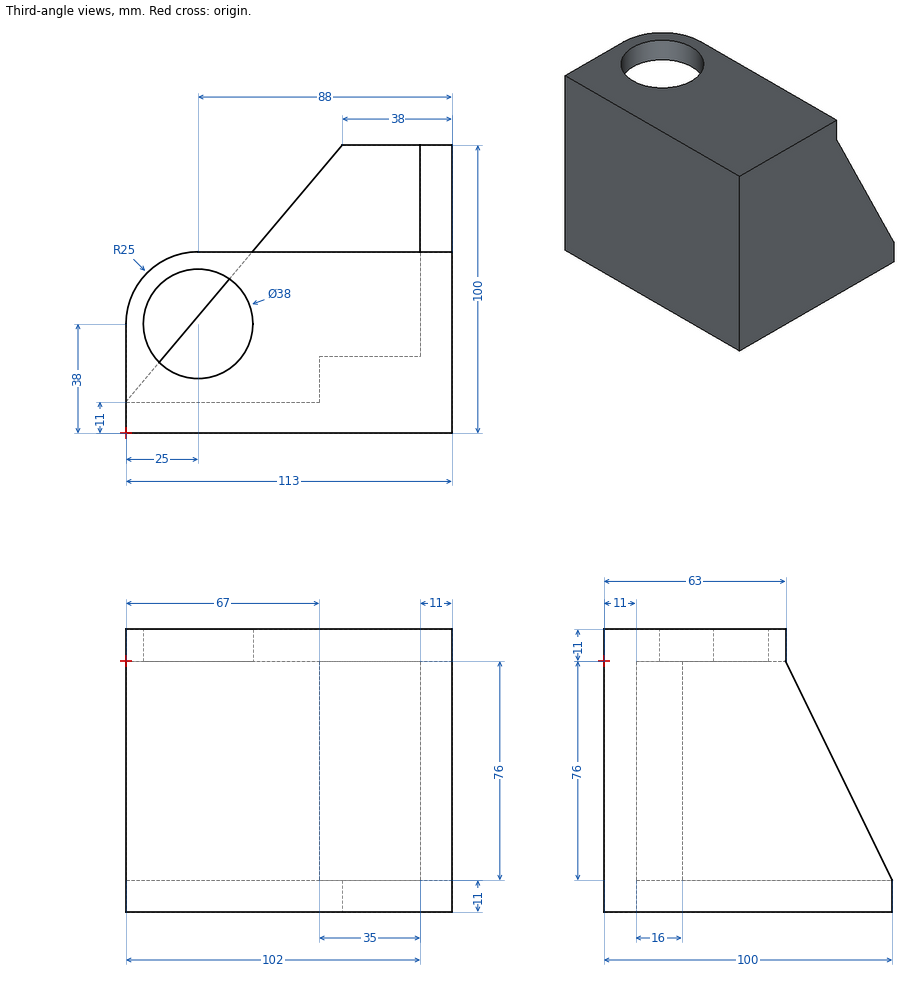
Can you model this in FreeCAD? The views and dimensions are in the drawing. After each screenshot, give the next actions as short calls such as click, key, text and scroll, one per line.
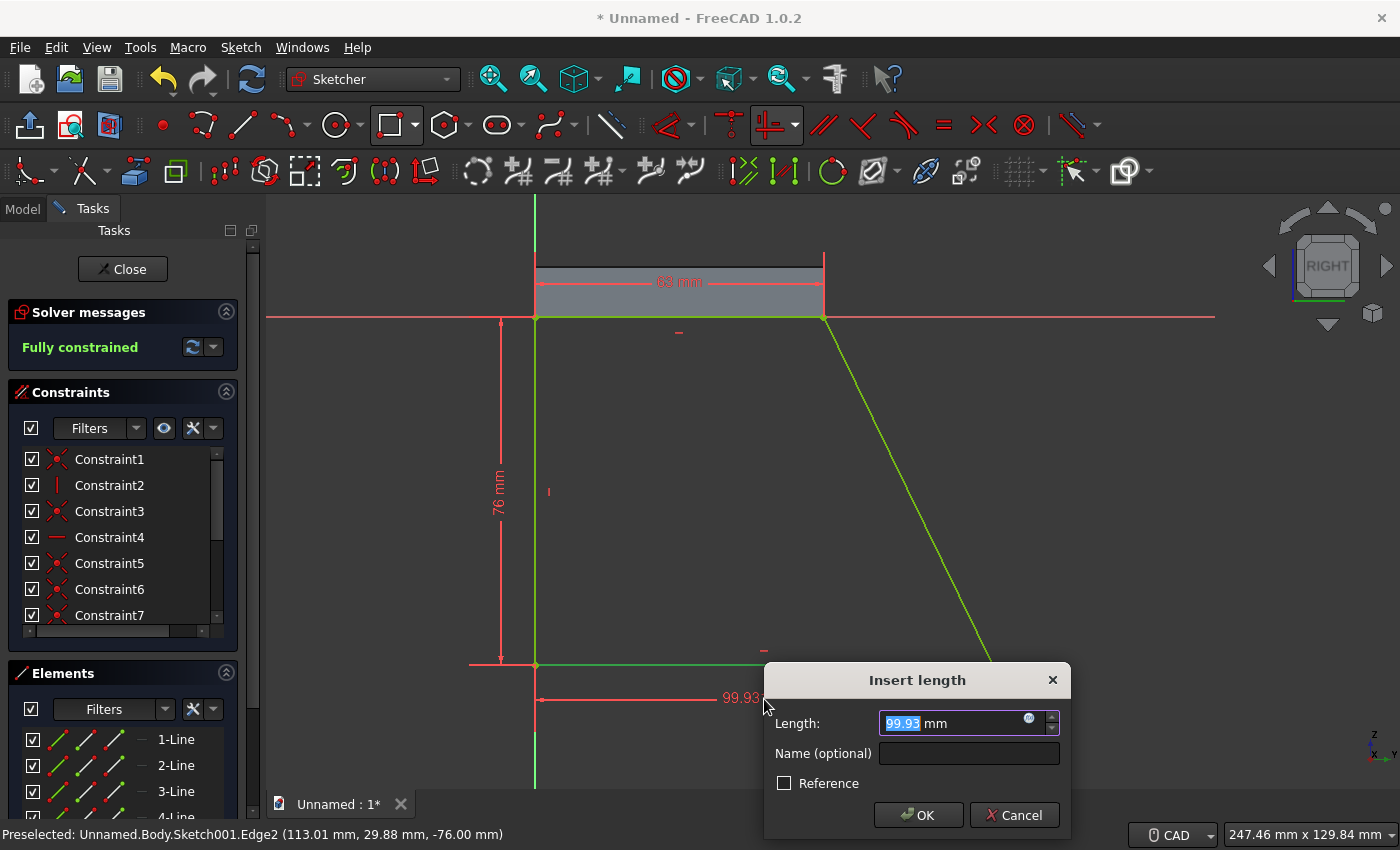
text(100)
key(Return)
key(Escape)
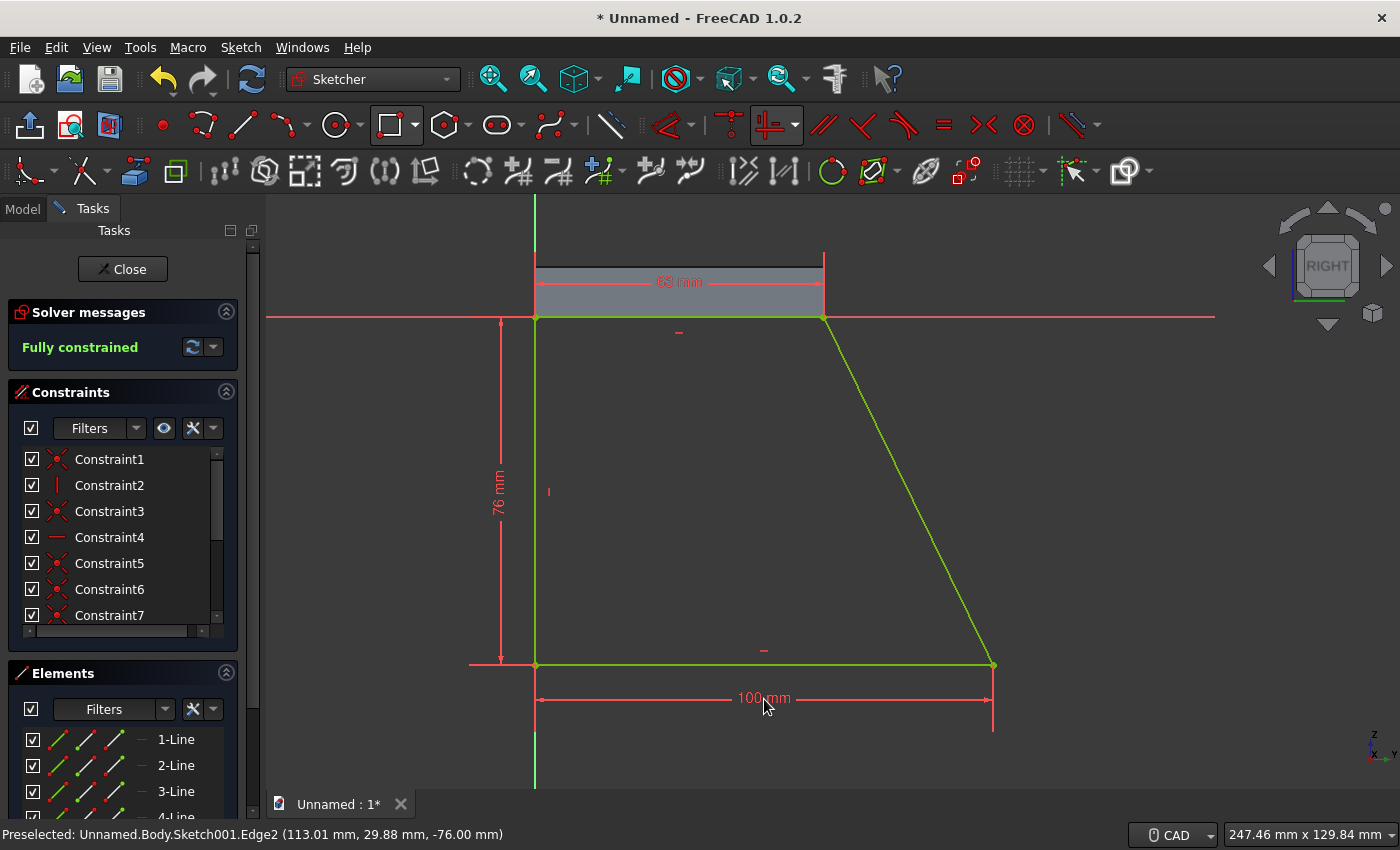
click(123, 269)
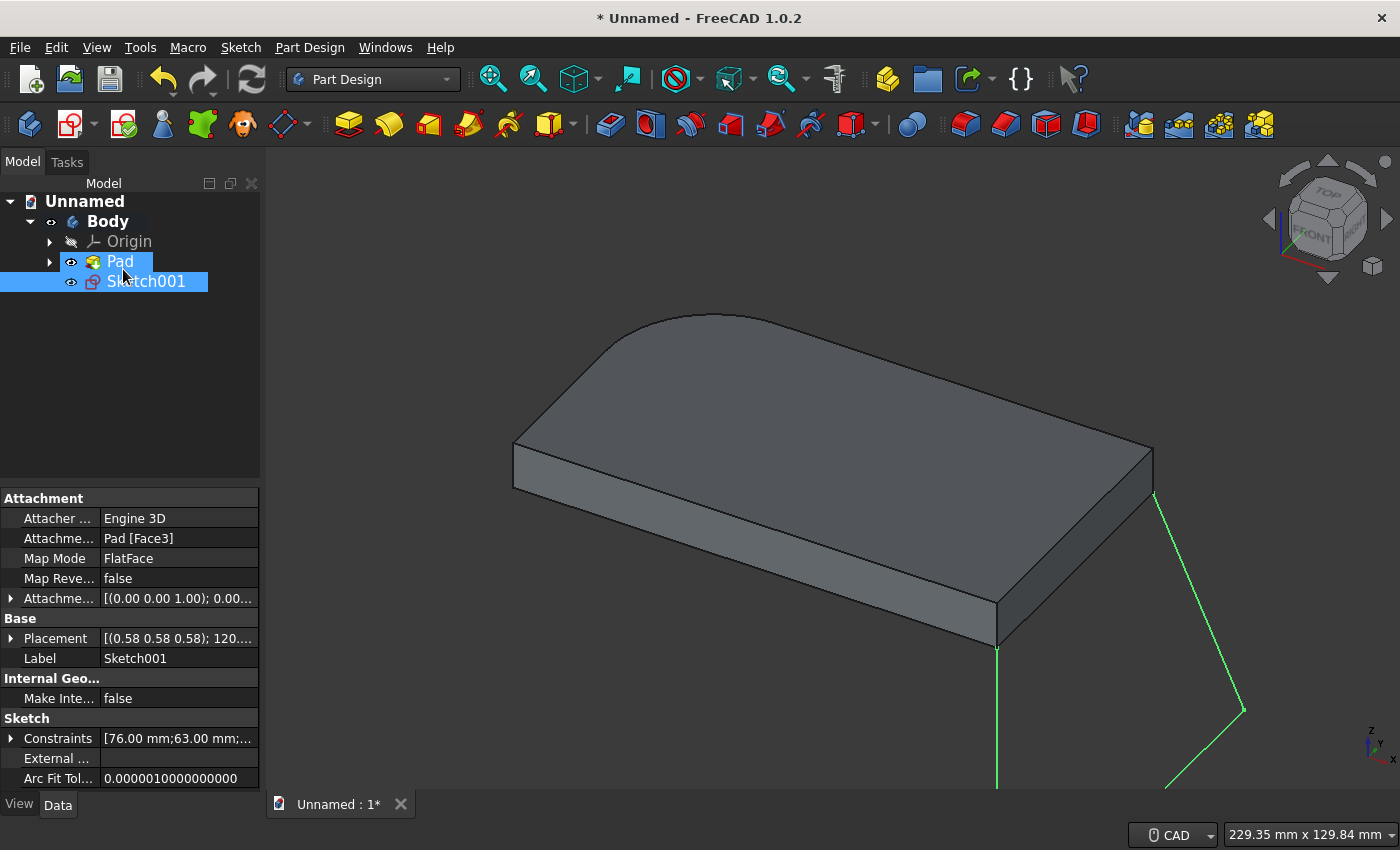
click(350, 124)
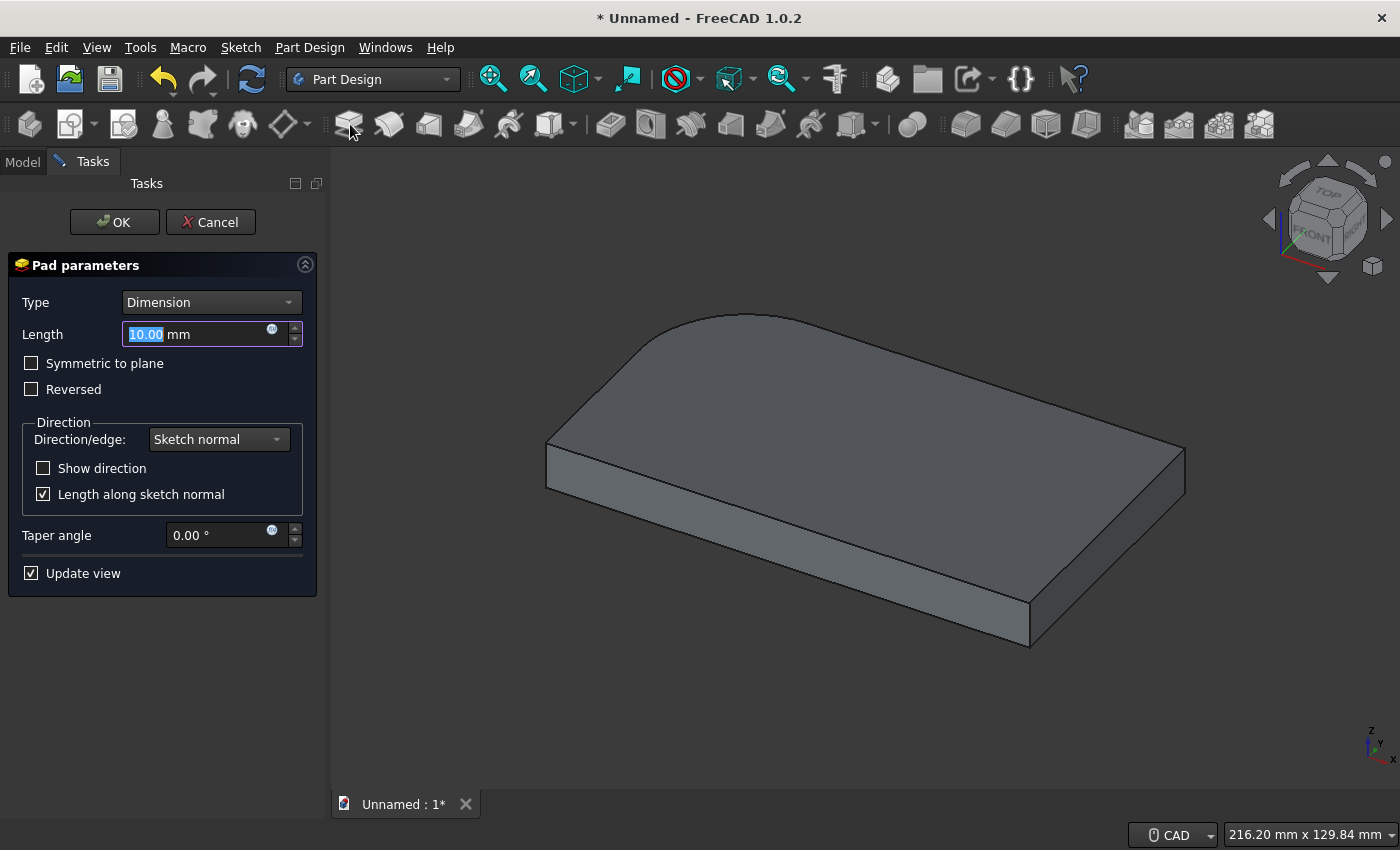
text(11)
key(Tab)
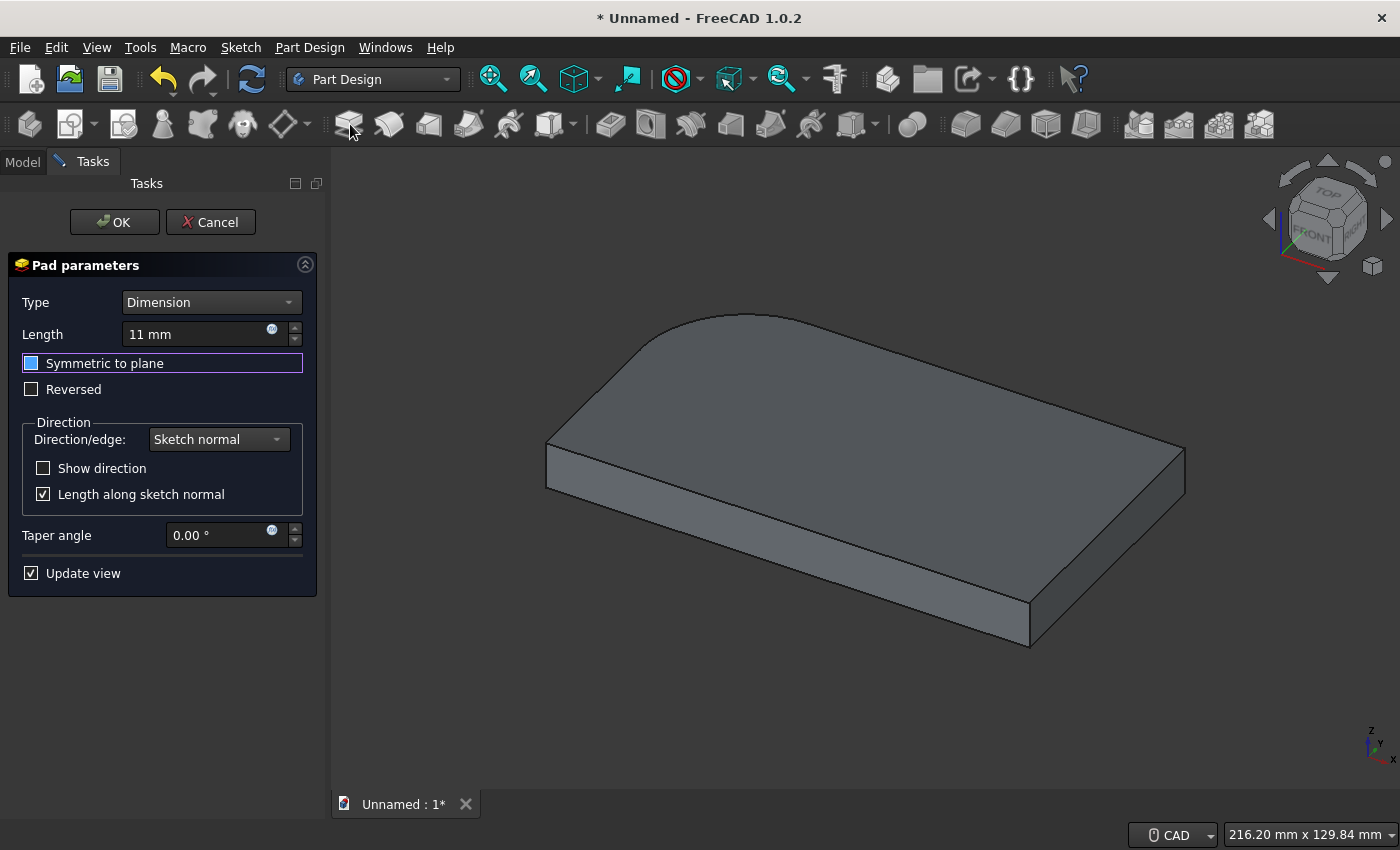
click(30, 389)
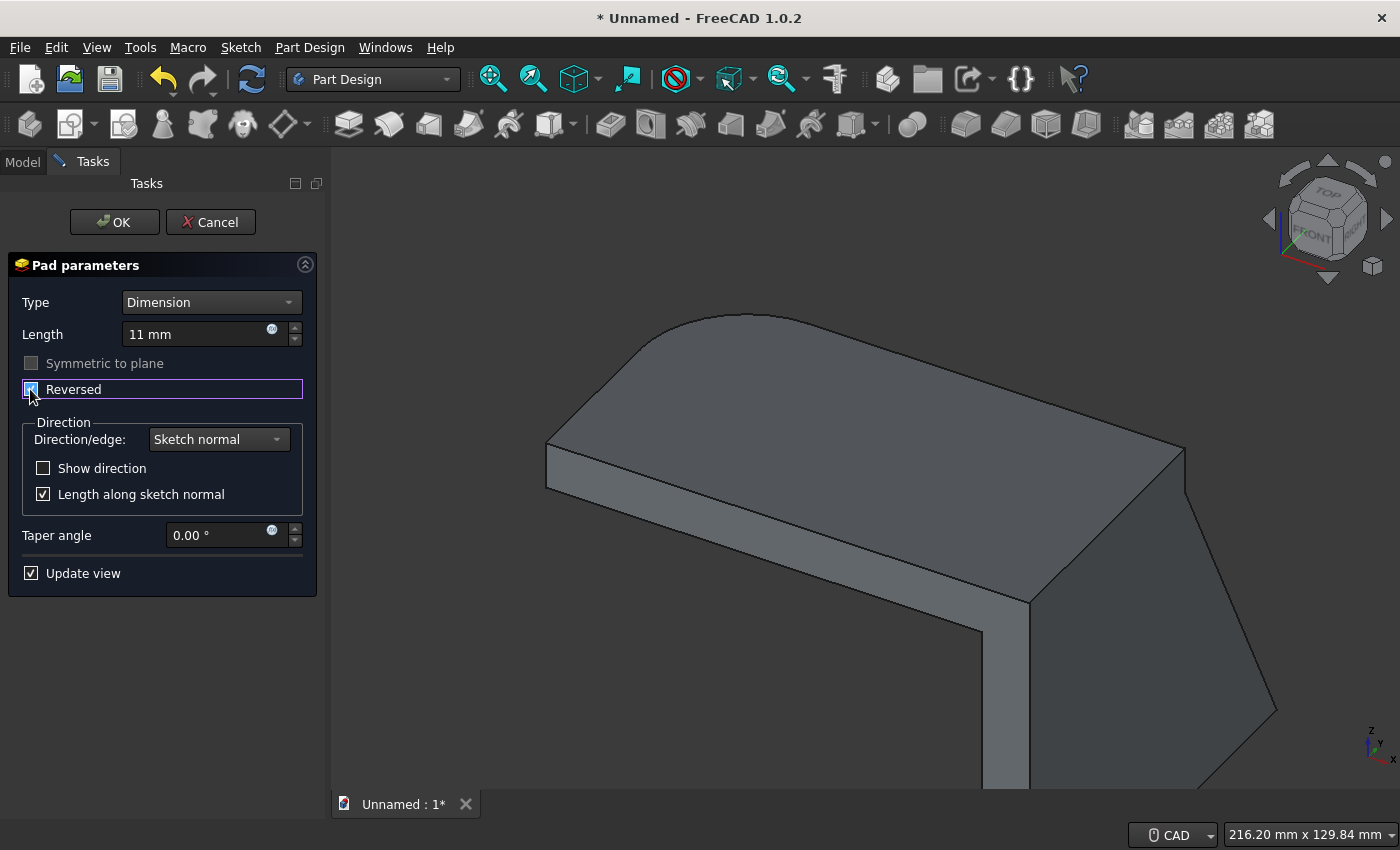
click(115, 222)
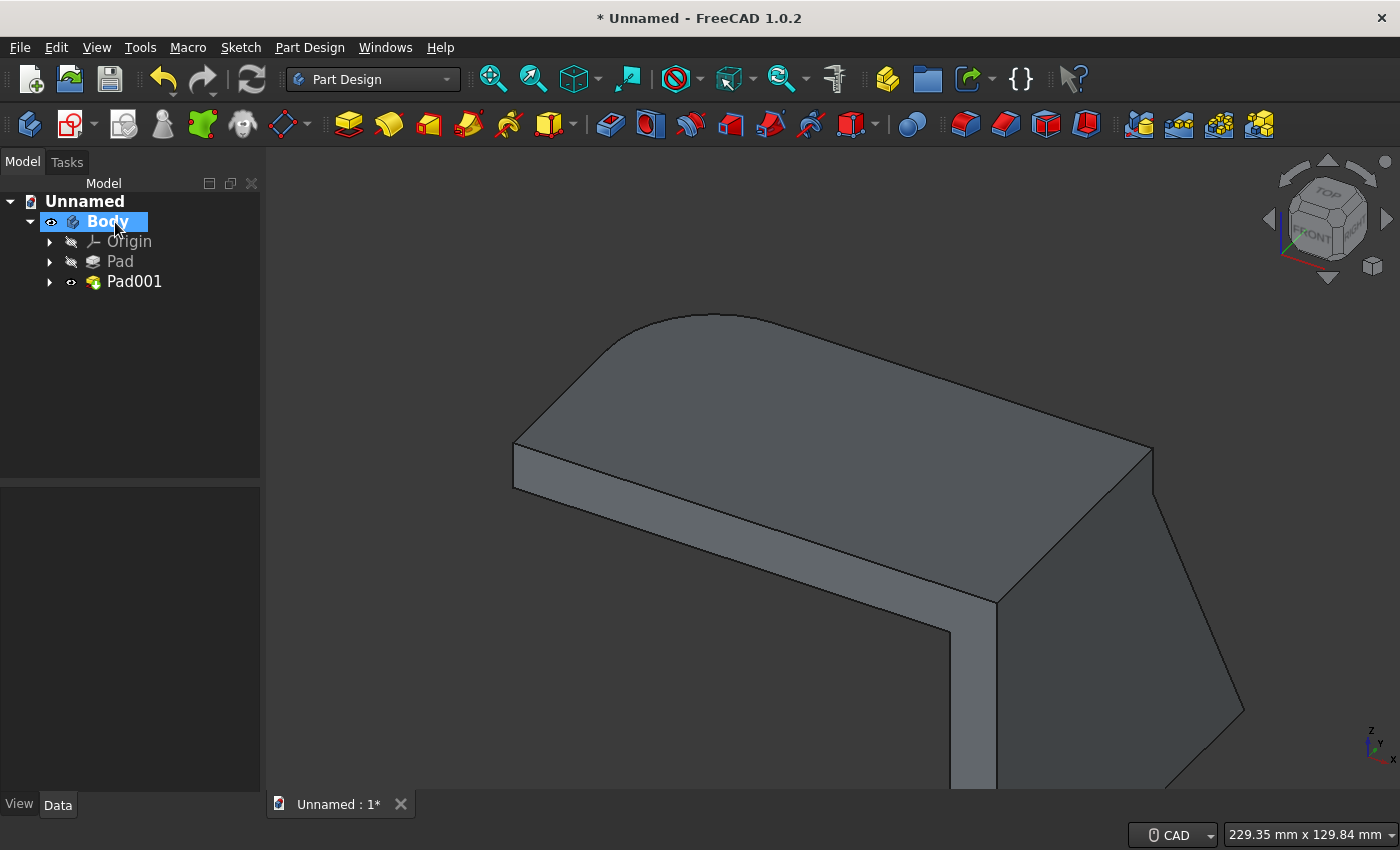
key(v)
key(f)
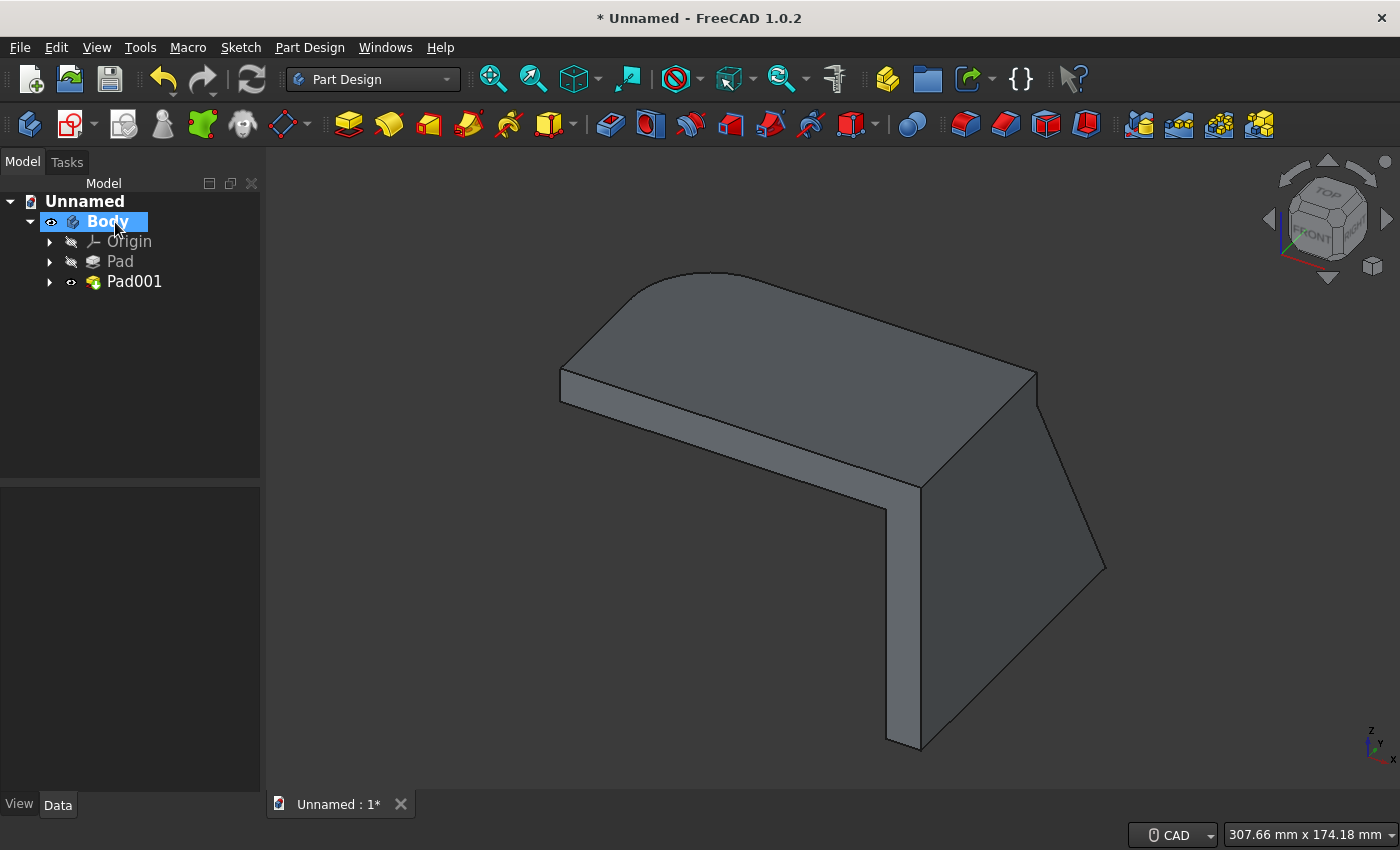
key(5)